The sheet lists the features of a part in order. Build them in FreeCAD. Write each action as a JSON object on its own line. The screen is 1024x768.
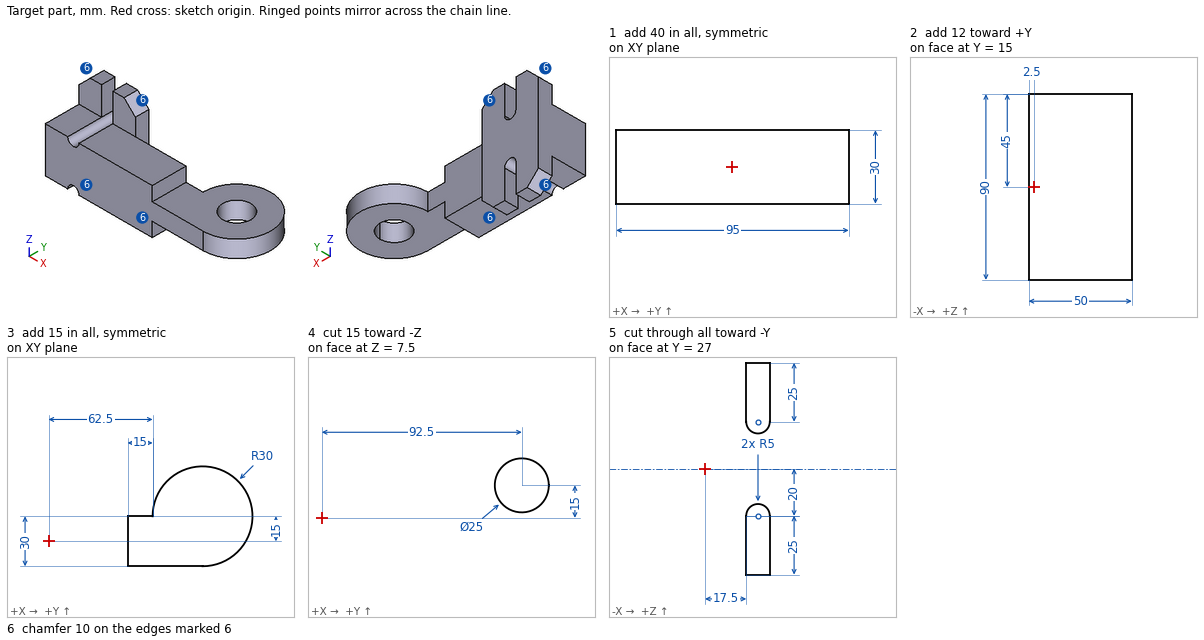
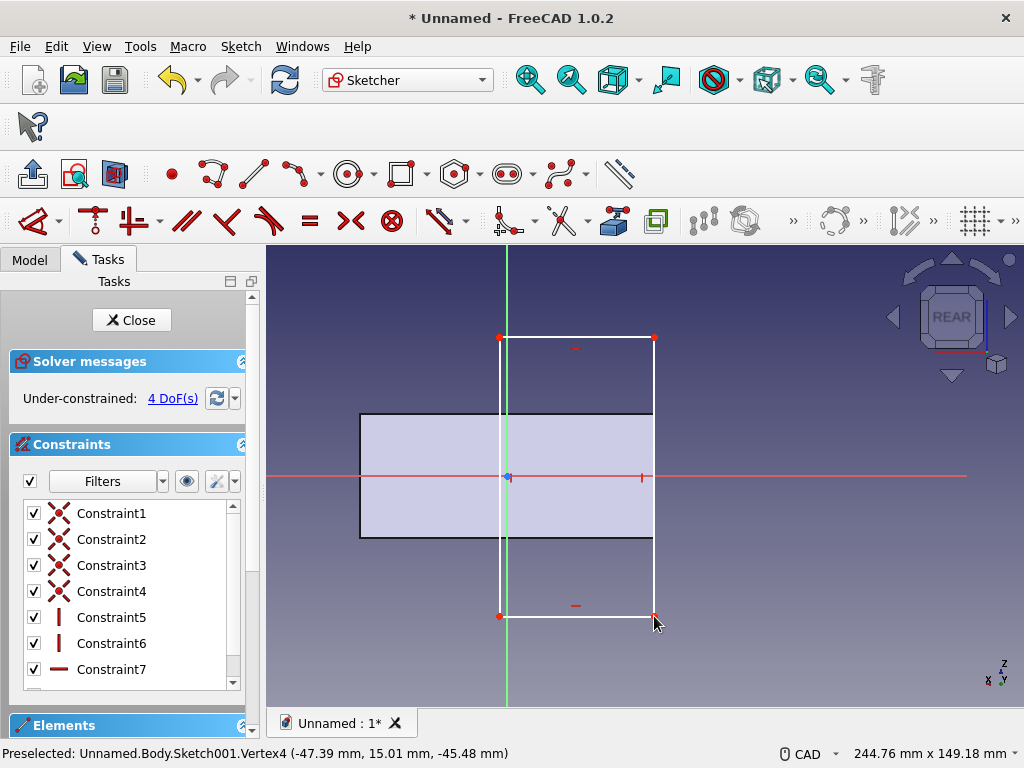
{"action": "left_click", "coordinate": [32, 222]}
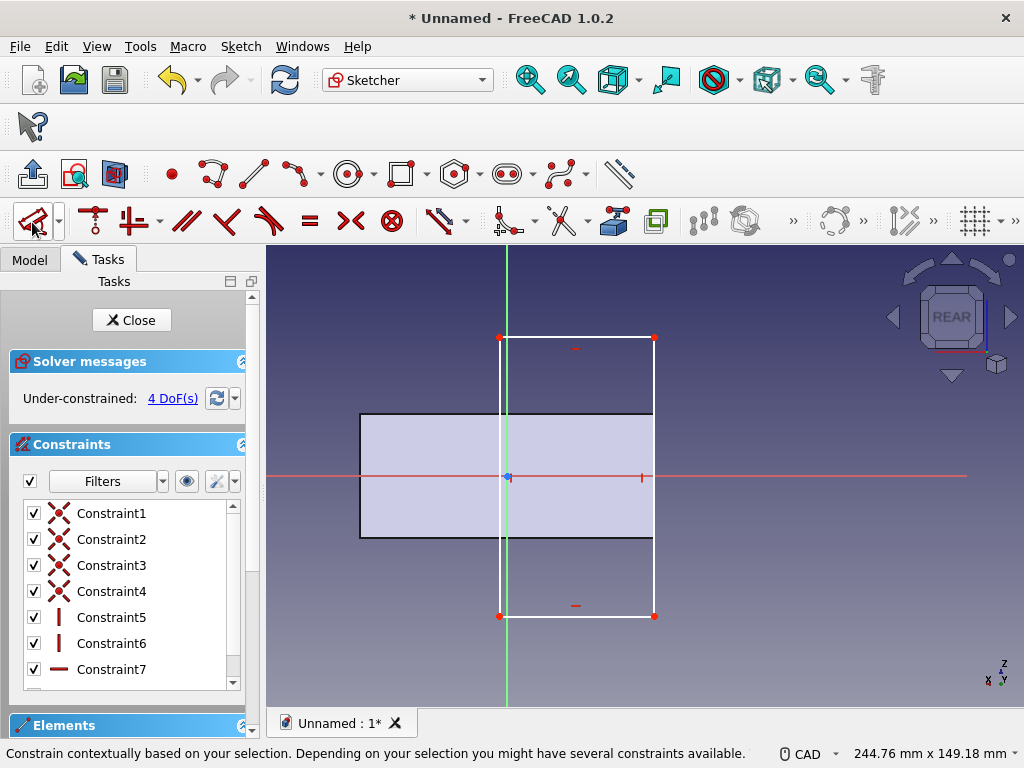
{"action": "scroll", "coordinate": [500, 421], "scroll_direction": "up", "scroll_amount": 4}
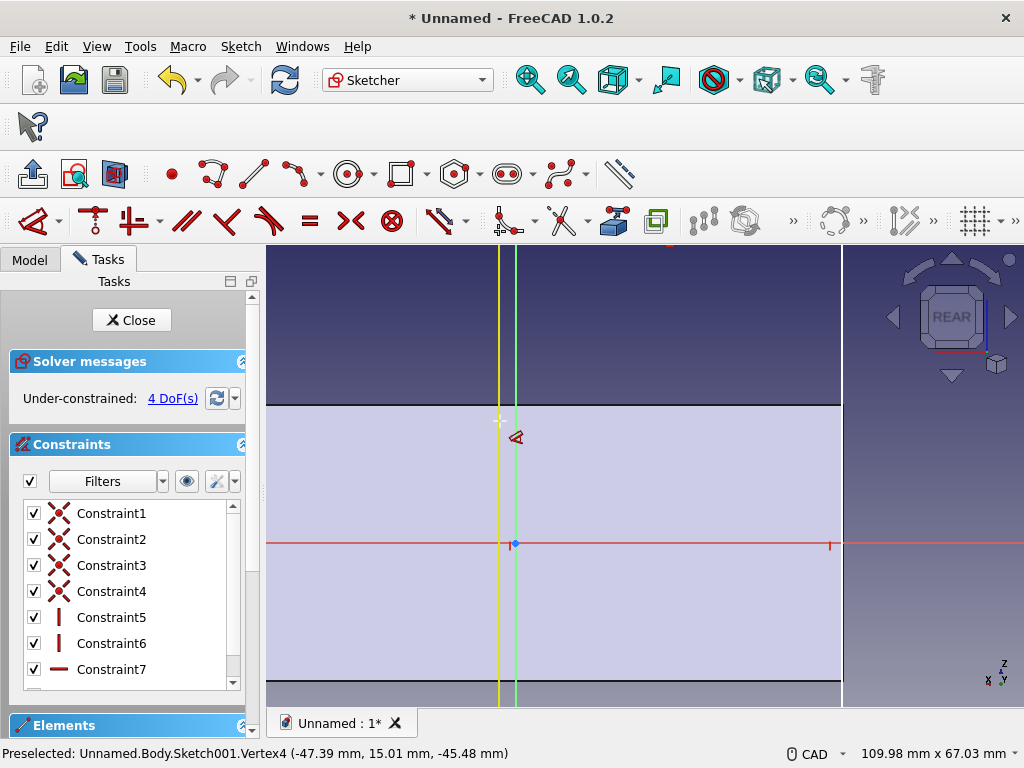
{"action": "left_click", "coordinate": [499, 421]}
{"action": "left_click", "coordinate": [465, 476]}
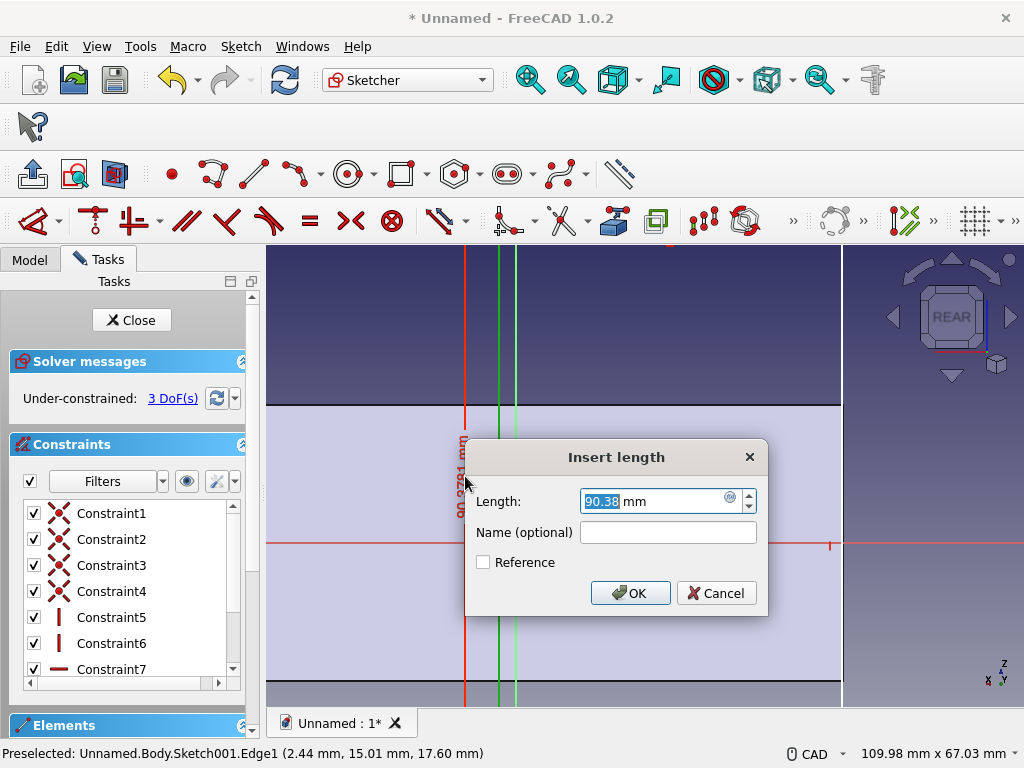
{"action": "type", "text": "90"}
{"action": "key", "text": "Return"}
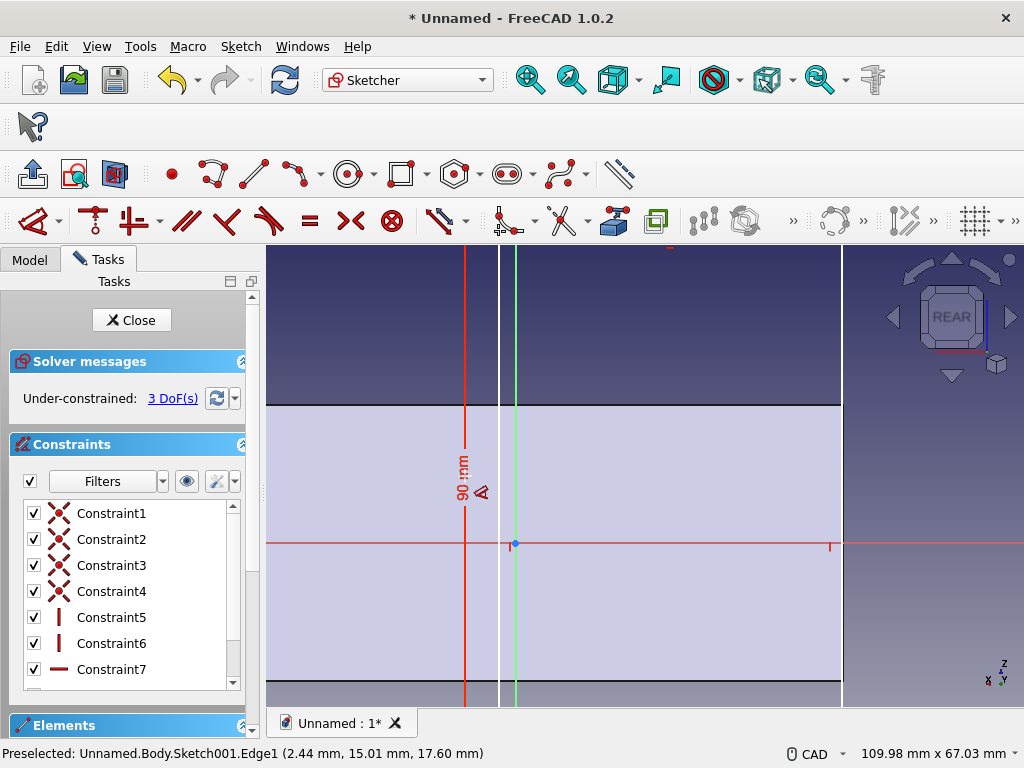
{"action": "scroll", "coordinate": [500, 421], "scroll_direction": "down", "scroll_amount": 4}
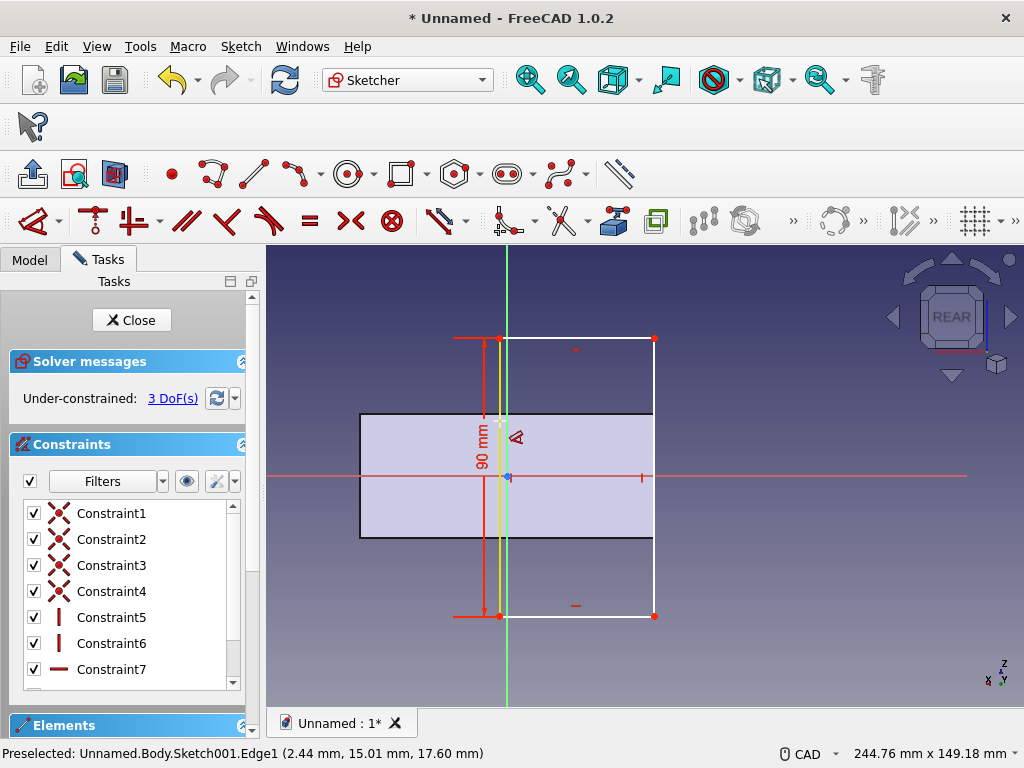
{"action": "left_click", "coordinate": [546, 617]}
{"action": "left_click", "coordinate": [577, 651]}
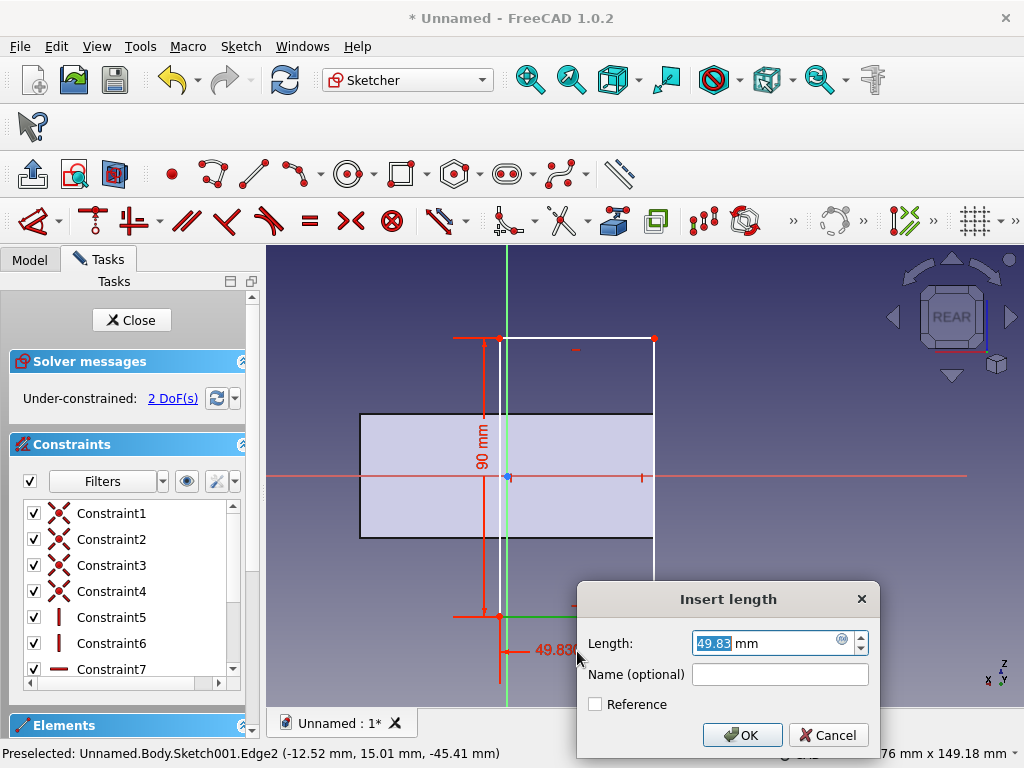
{"action": "type", "text": "50"}
{"action": "key", "text": "Return"}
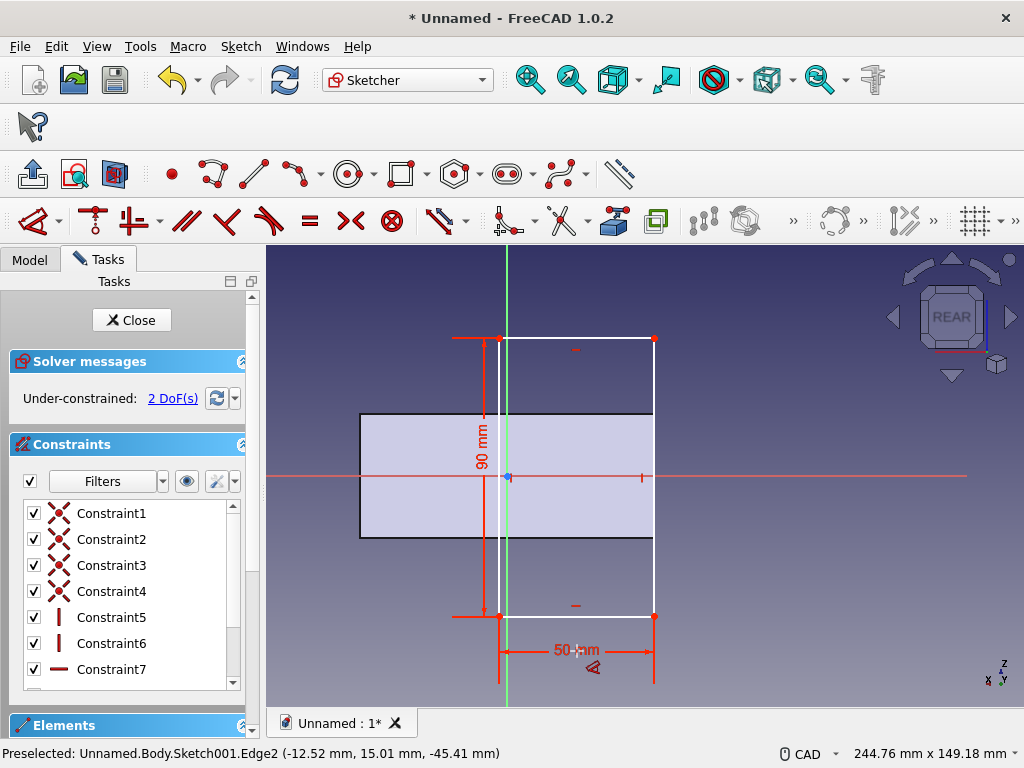
{"action": "left_click", "coordinate": [499, 338]}
{"action": "left_click", "coordinate": [465, 407]}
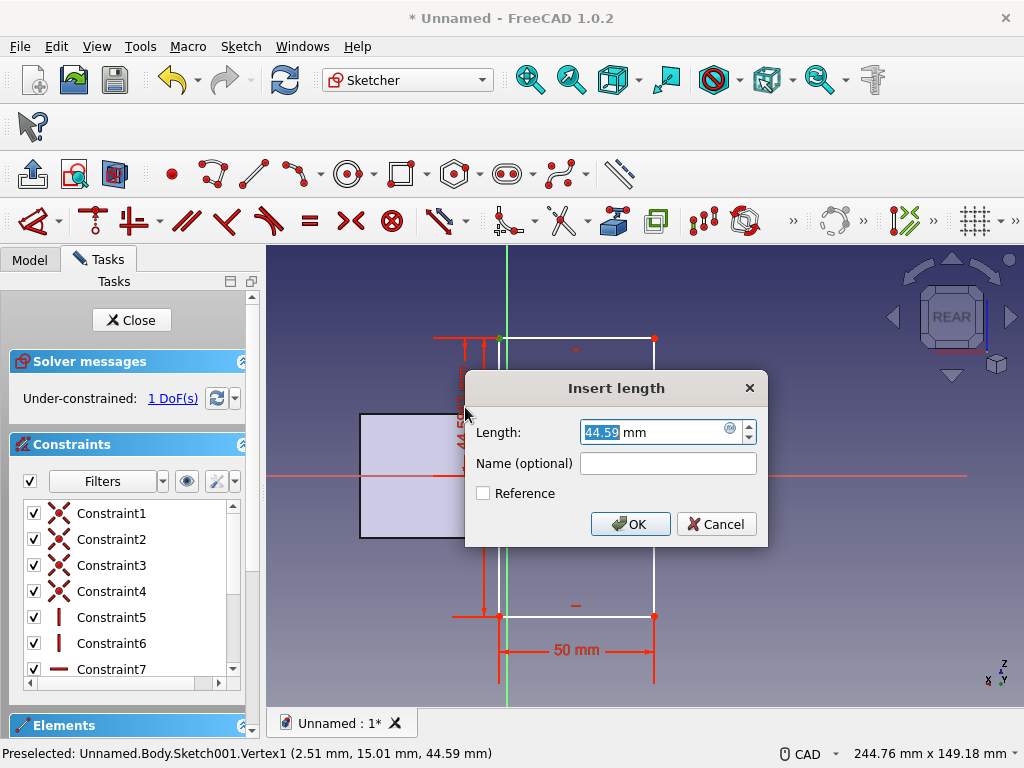
{"action": "type", "text": "45"}
{"action": "key", "text": "Return"}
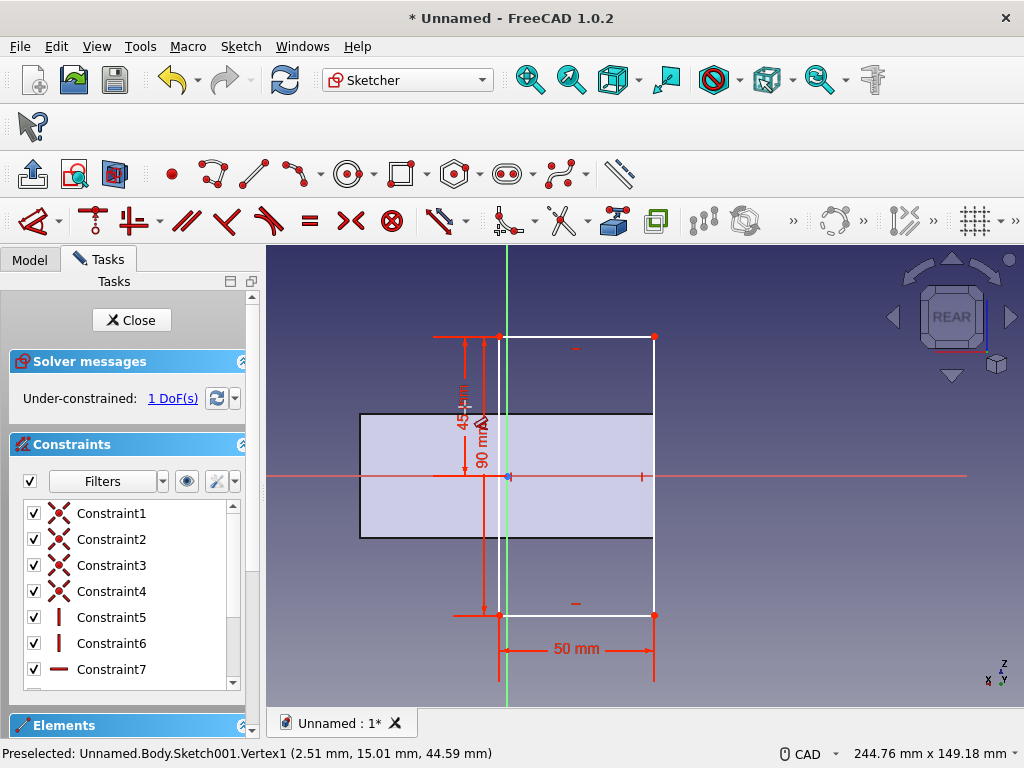
{"action": "scroll", "coordinate": [499, 337], "scroll_direction": "up", "scroll_amount": 9}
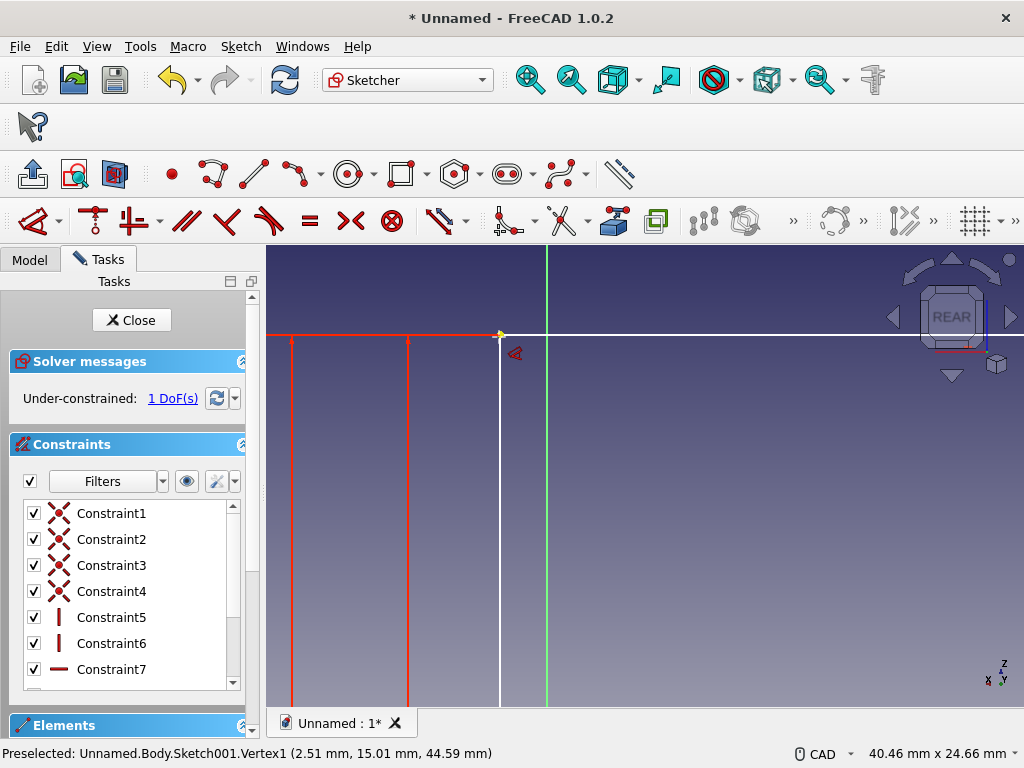
{"action": "left_click", "coordinate": [500, 335]}
{"action": "left_click", "coordinate": [524, 301]}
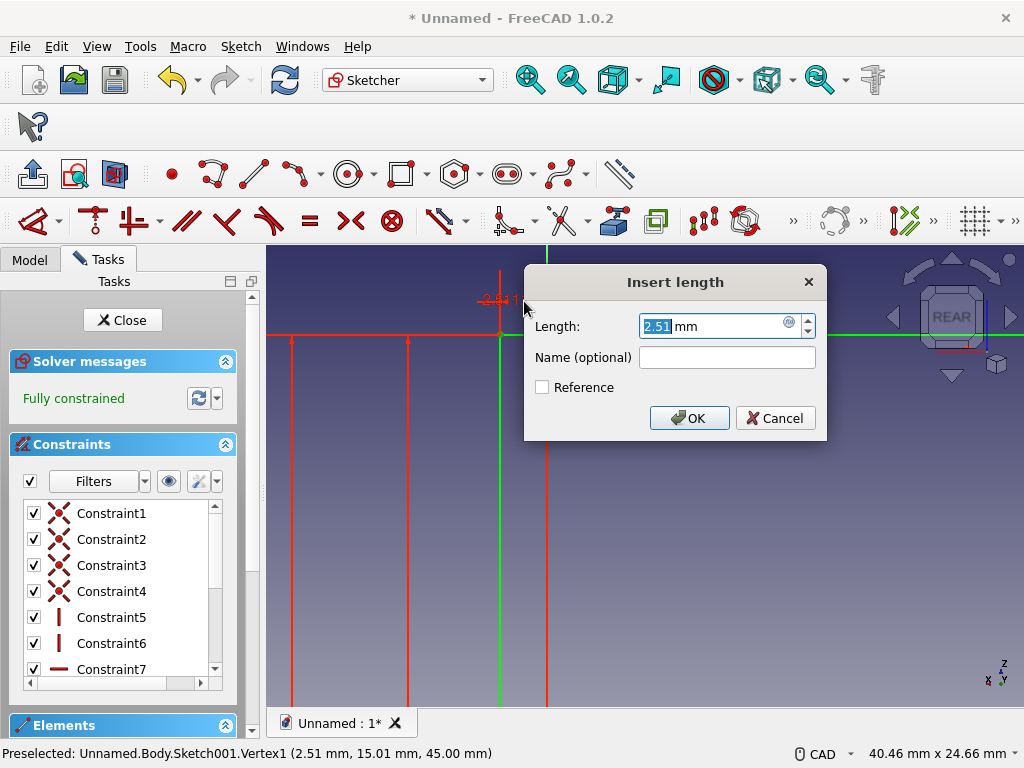
{"action": "type", "text": "2.5"}
{"action": "key", "text": "Return"}
{"action": "key", "text": "Escape"}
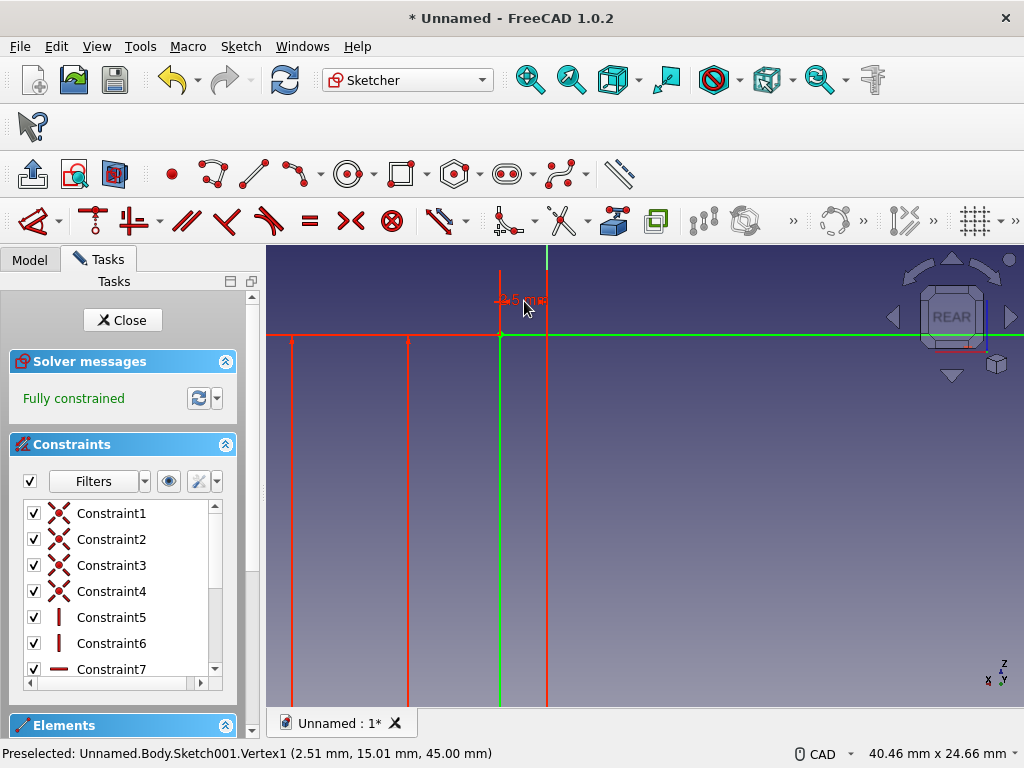
{"action": "left_click", "coordinate": [123, 320]}